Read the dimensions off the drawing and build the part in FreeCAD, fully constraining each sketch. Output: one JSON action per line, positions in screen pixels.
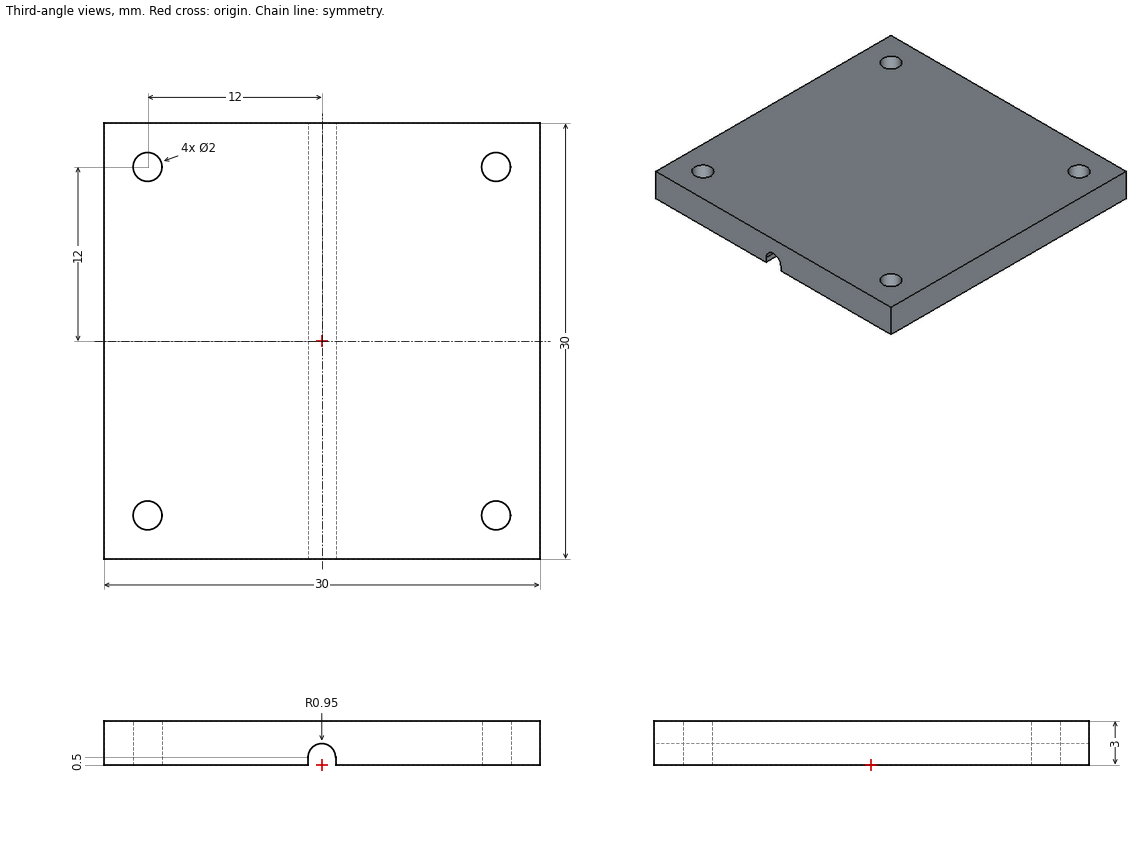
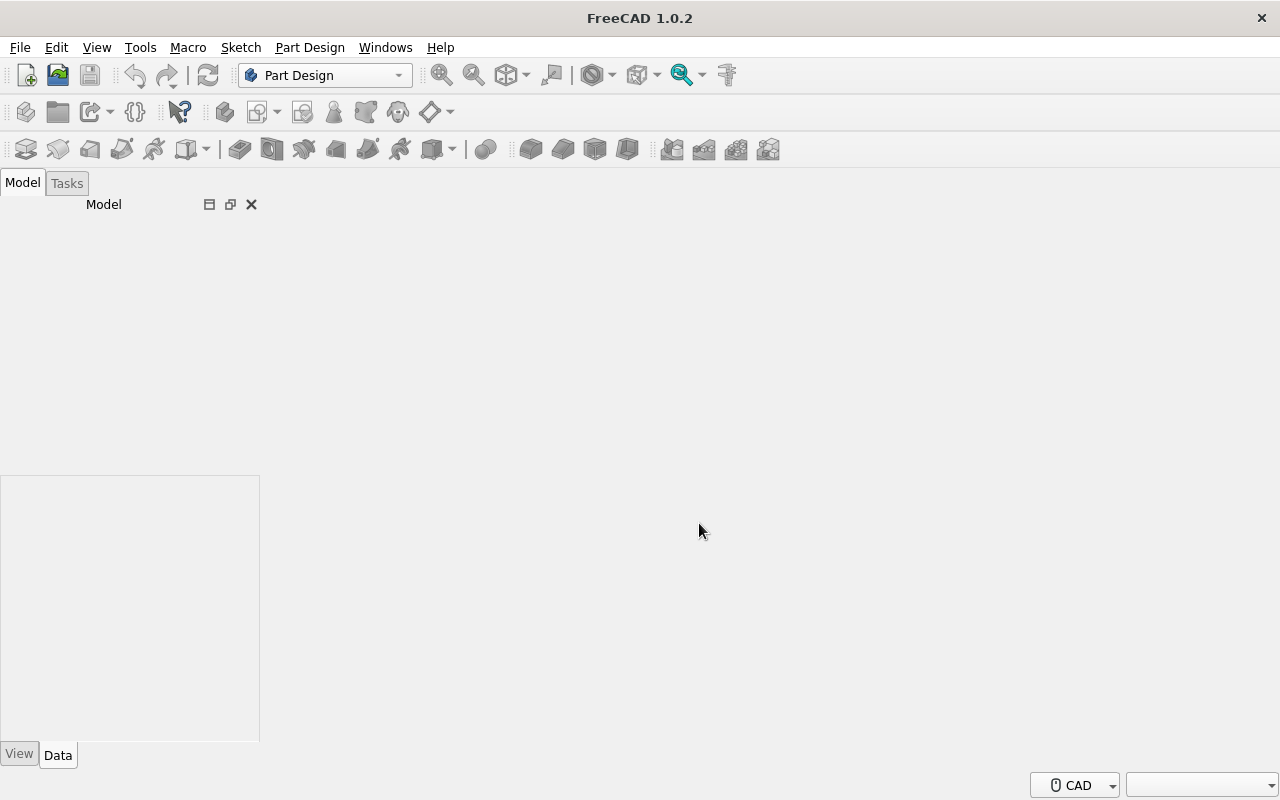
{"action": "left_click", "coordinate": [26, 76]}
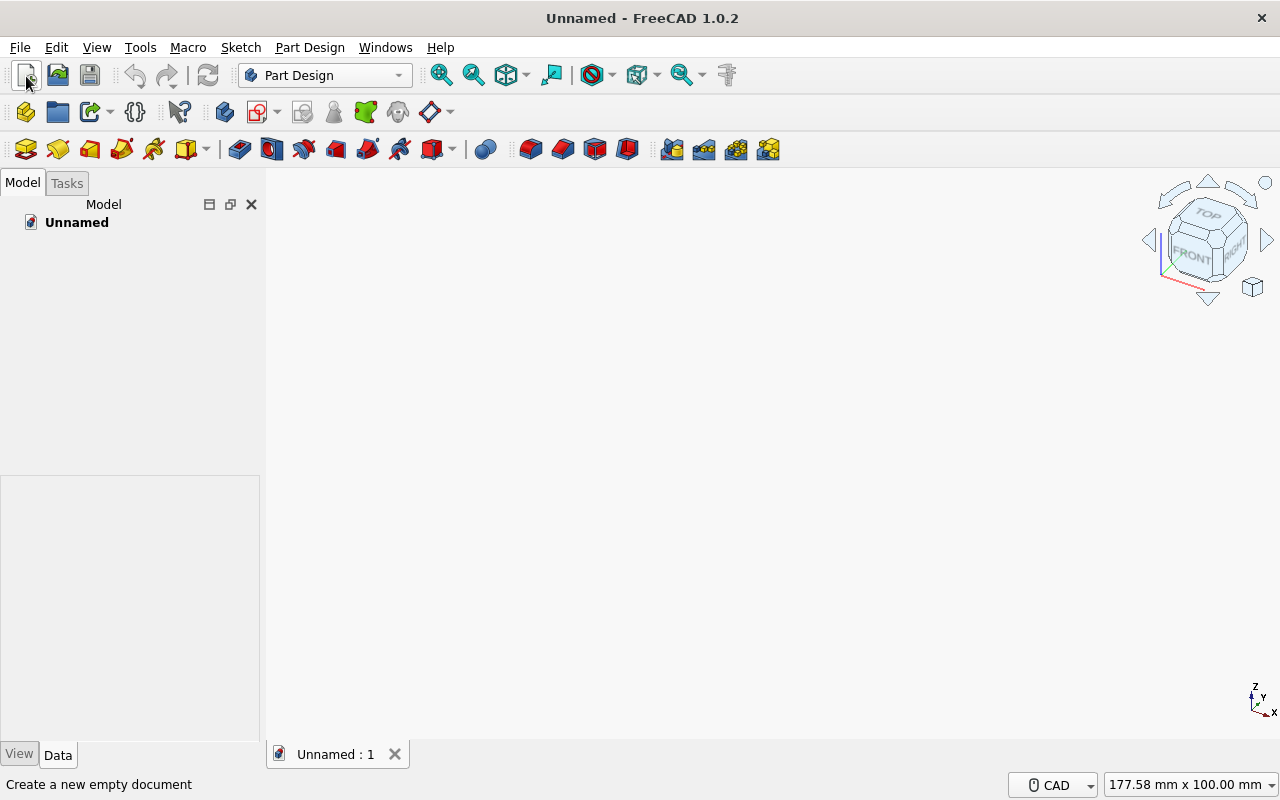
{"action": "left_click", "coordinate": [258, 112]}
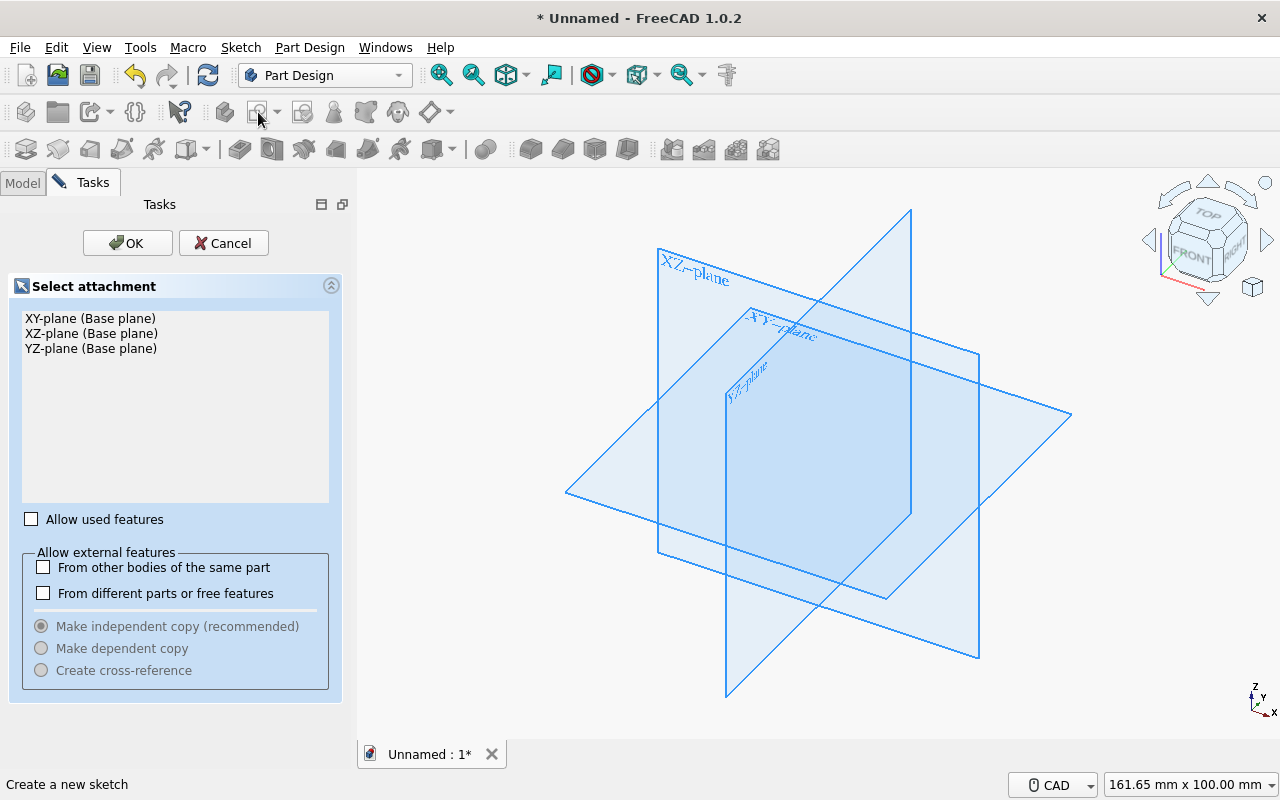
{"action": "left_click", "coordinate": [82, 318]}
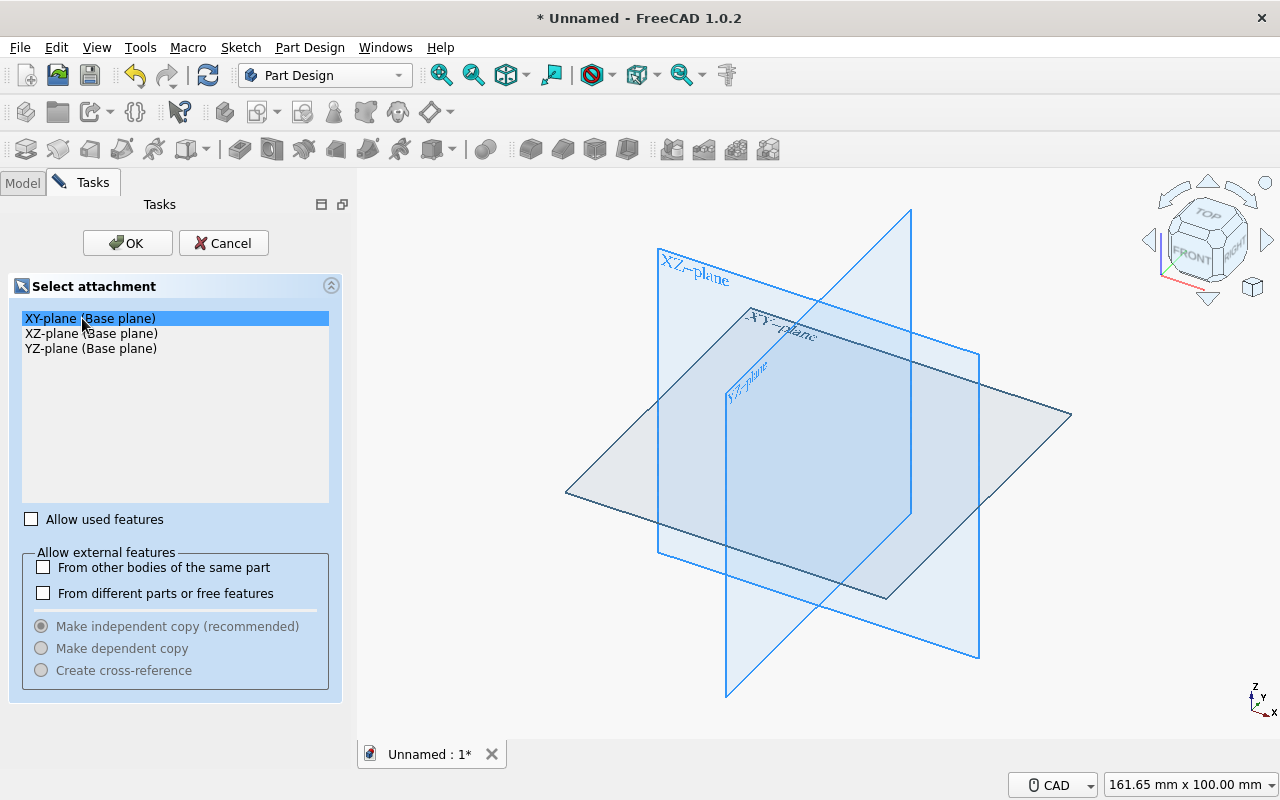
{"action": "left_click", "coordinate": [128, 243]}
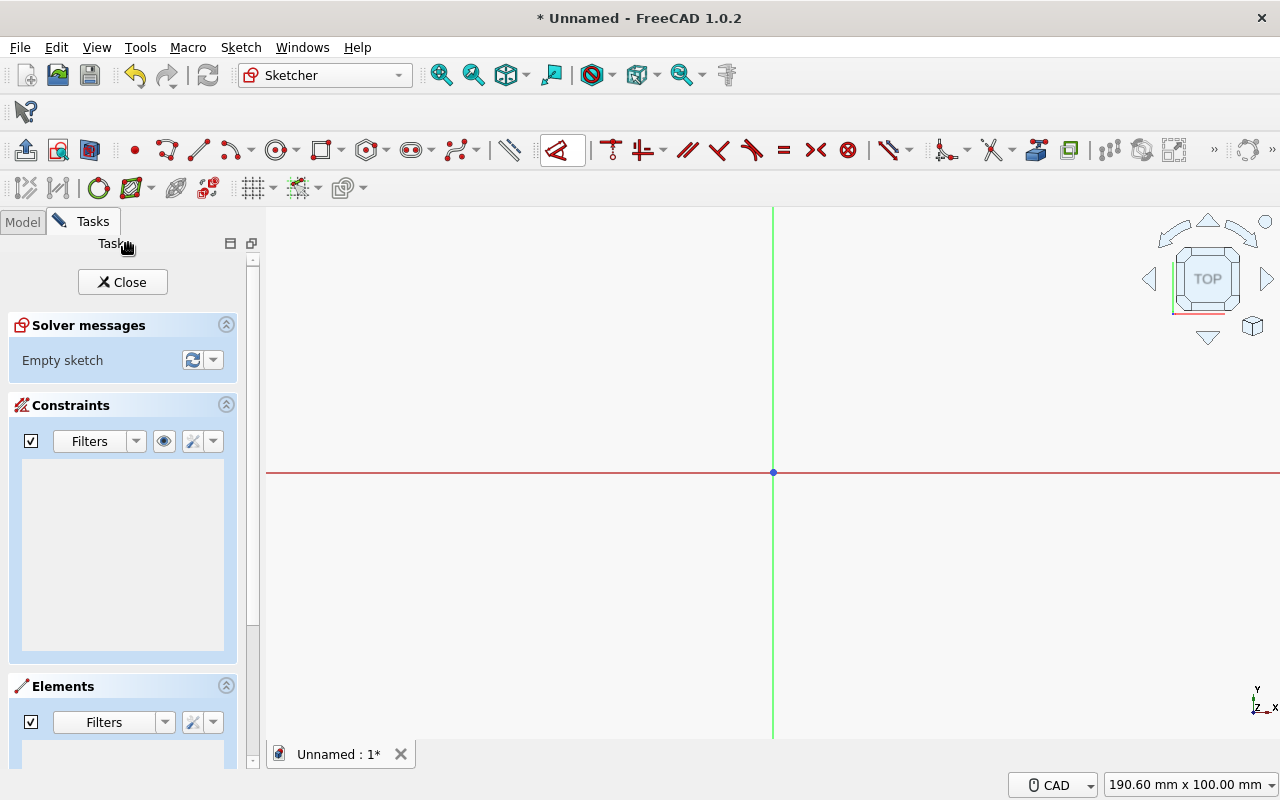
{"action": "scroll", "coordinate": [829, 473], "scroll_direction": "up", "scroll_amount": 4}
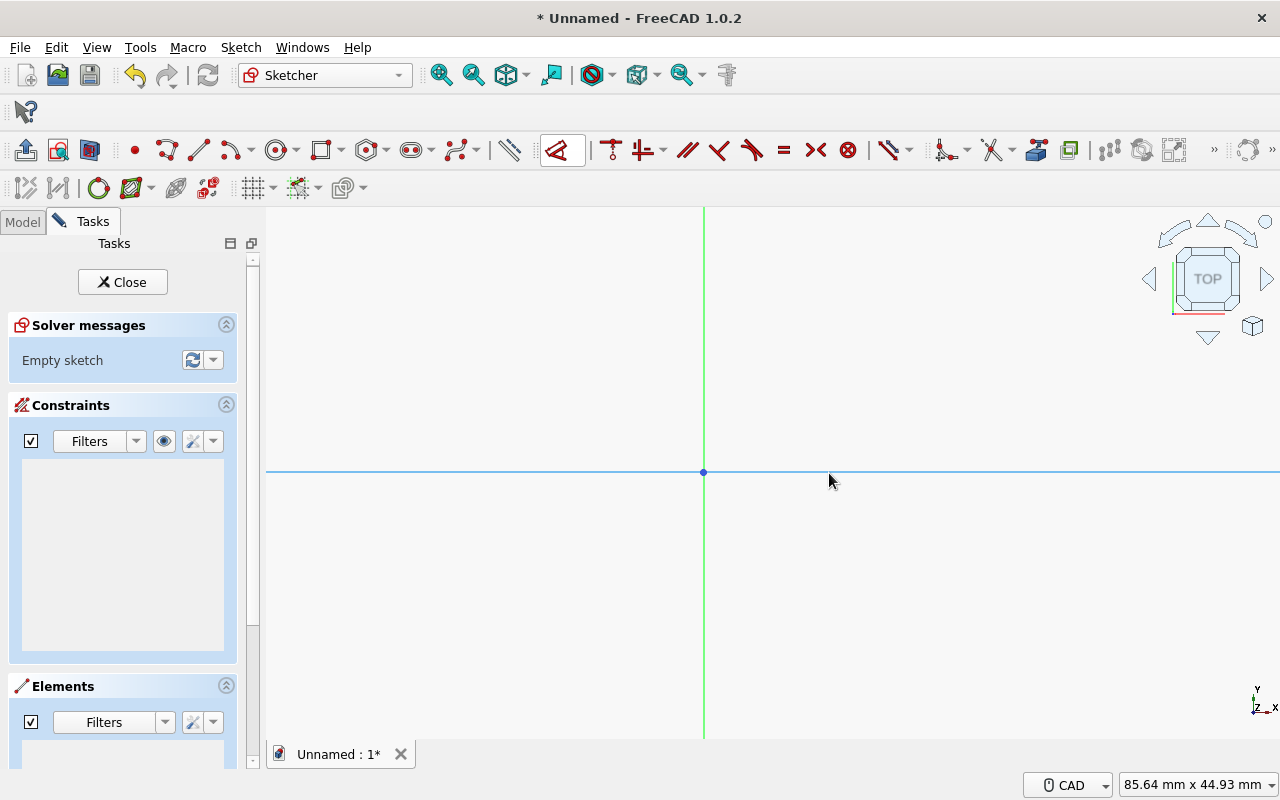
{"action": "left_click", "coordinate": [344, 150]}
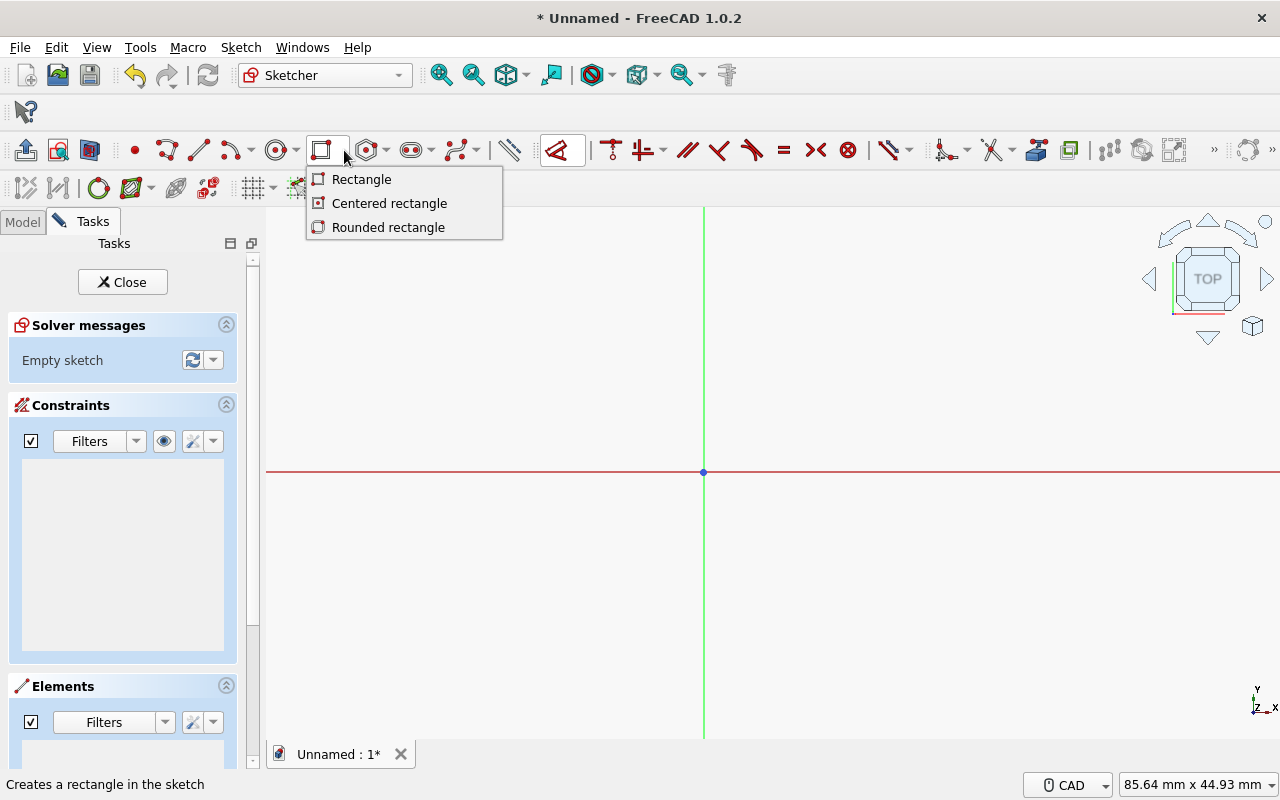
{"action": "left_click", "coordinate": [404, 203]}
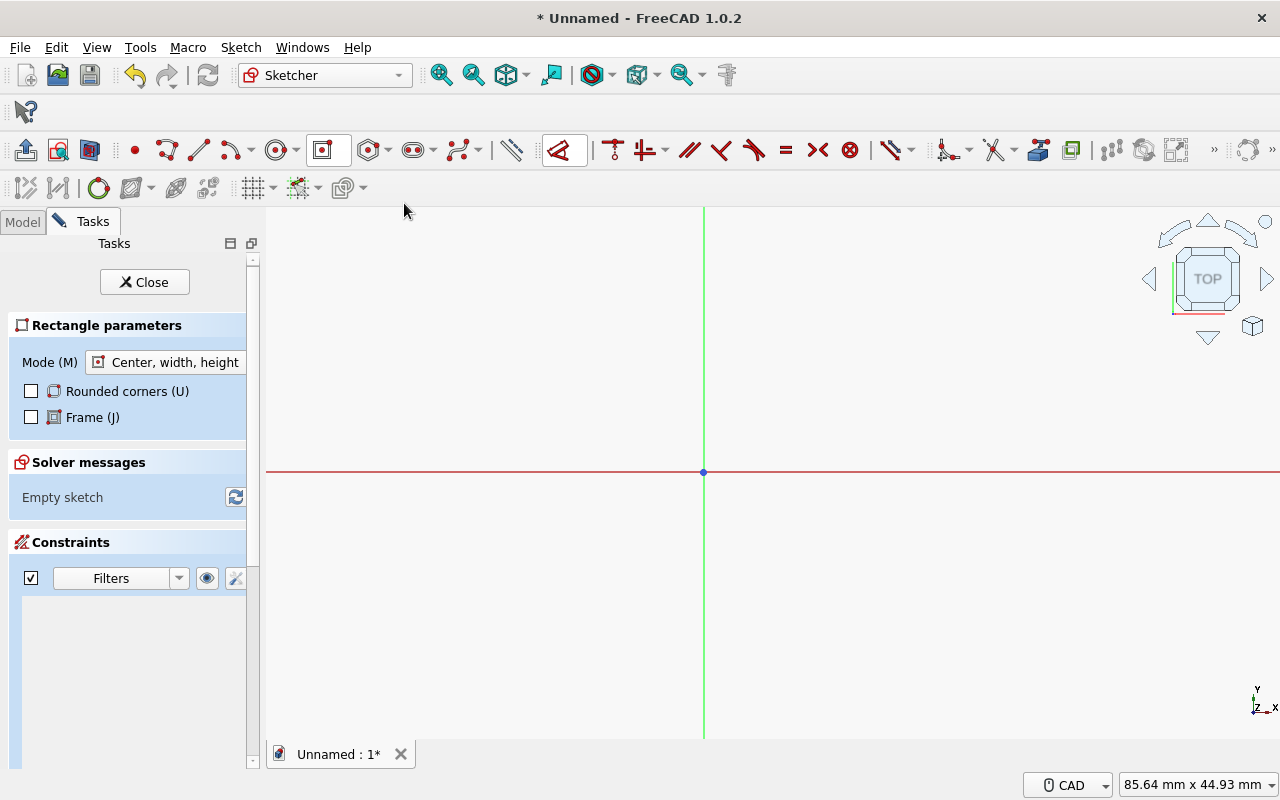
{"action": "left_click", "coordinate": [704, 472]}
{"action": "mouse_move", "coordinate": [881, 295]}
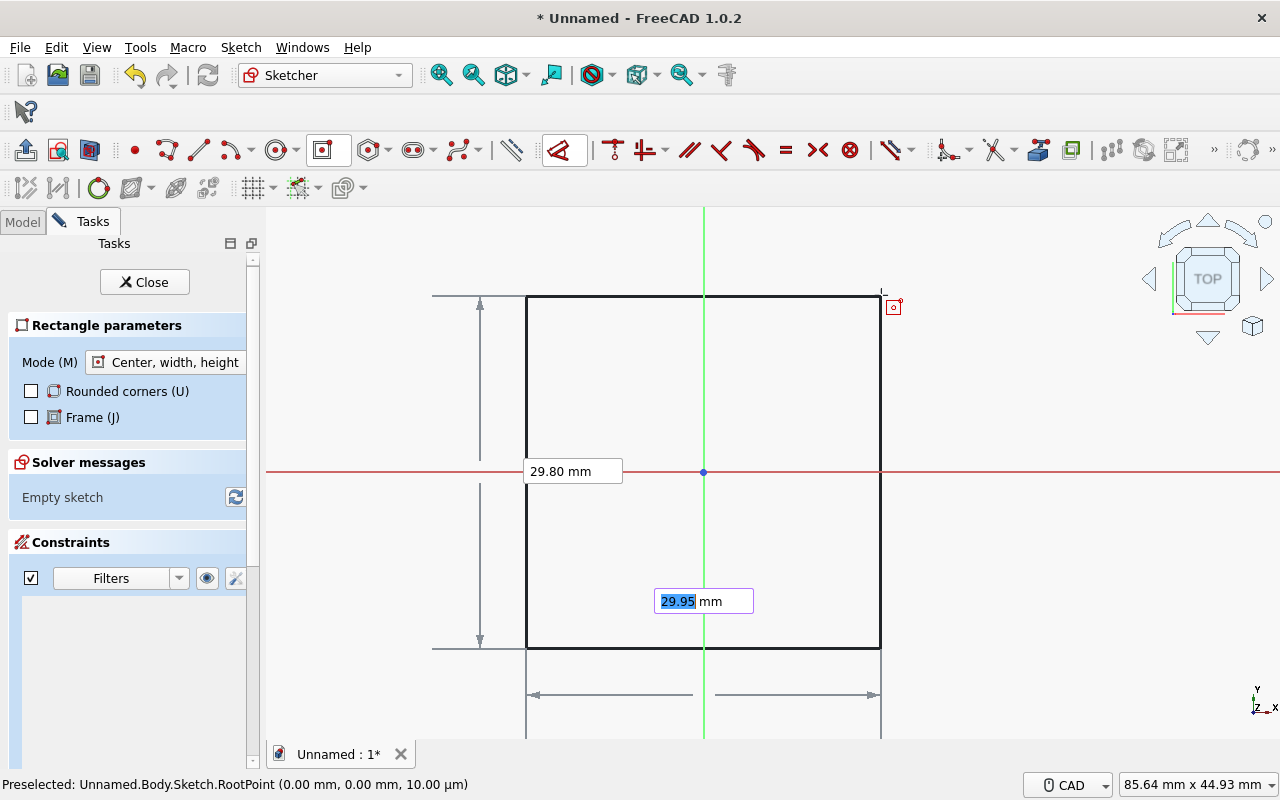
{"action": "type", "text": "30"}
{"action": "key", "text": "Tab"}
{"action": "type", "text": "30"}
{"action": "key", "text": "Return"}
{"action": "key", "text": "Escape"}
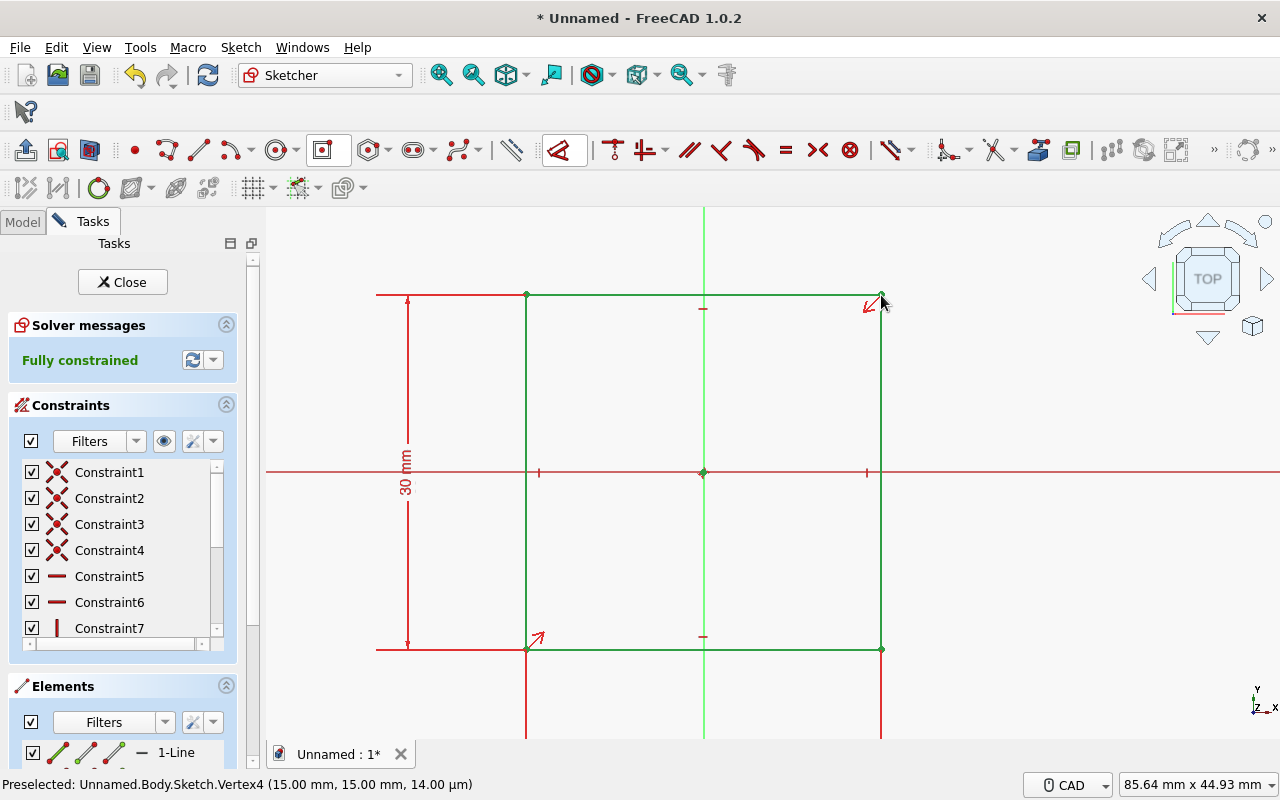
{"action": "left_click", "coordinate": [123, 282]}